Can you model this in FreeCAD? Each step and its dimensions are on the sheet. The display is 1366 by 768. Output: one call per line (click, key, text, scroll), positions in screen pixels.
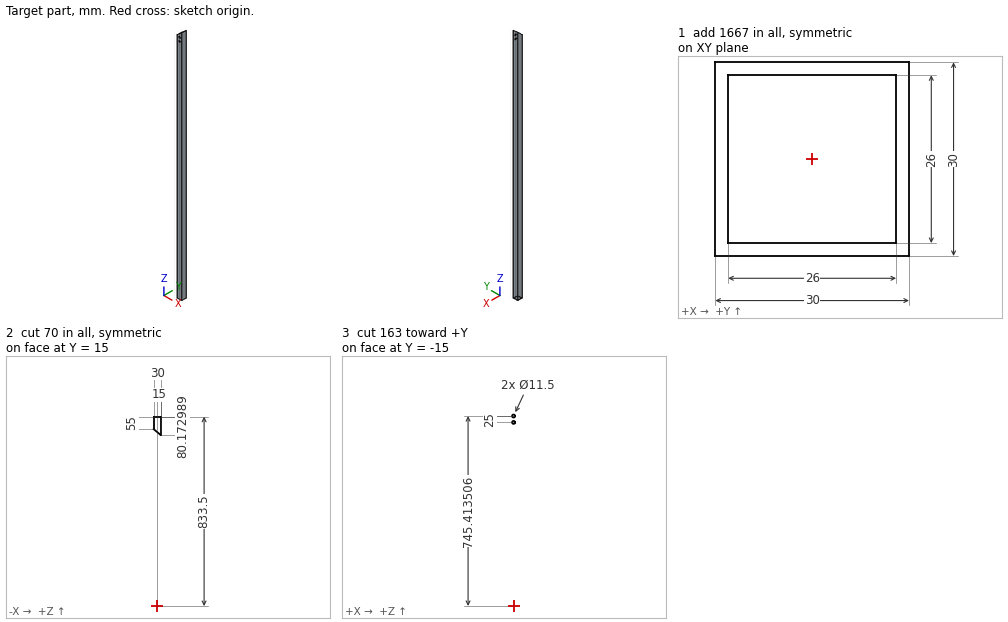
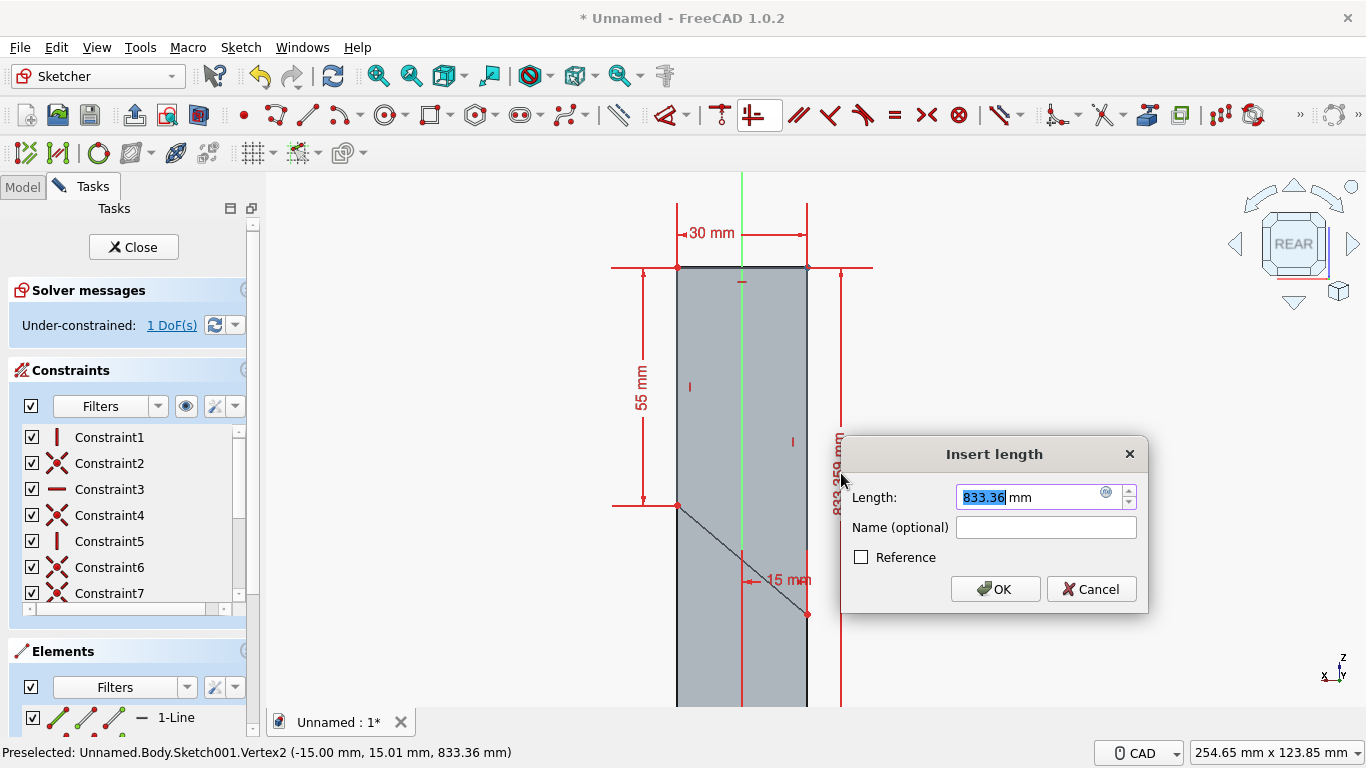
text(833.5)
key(Return)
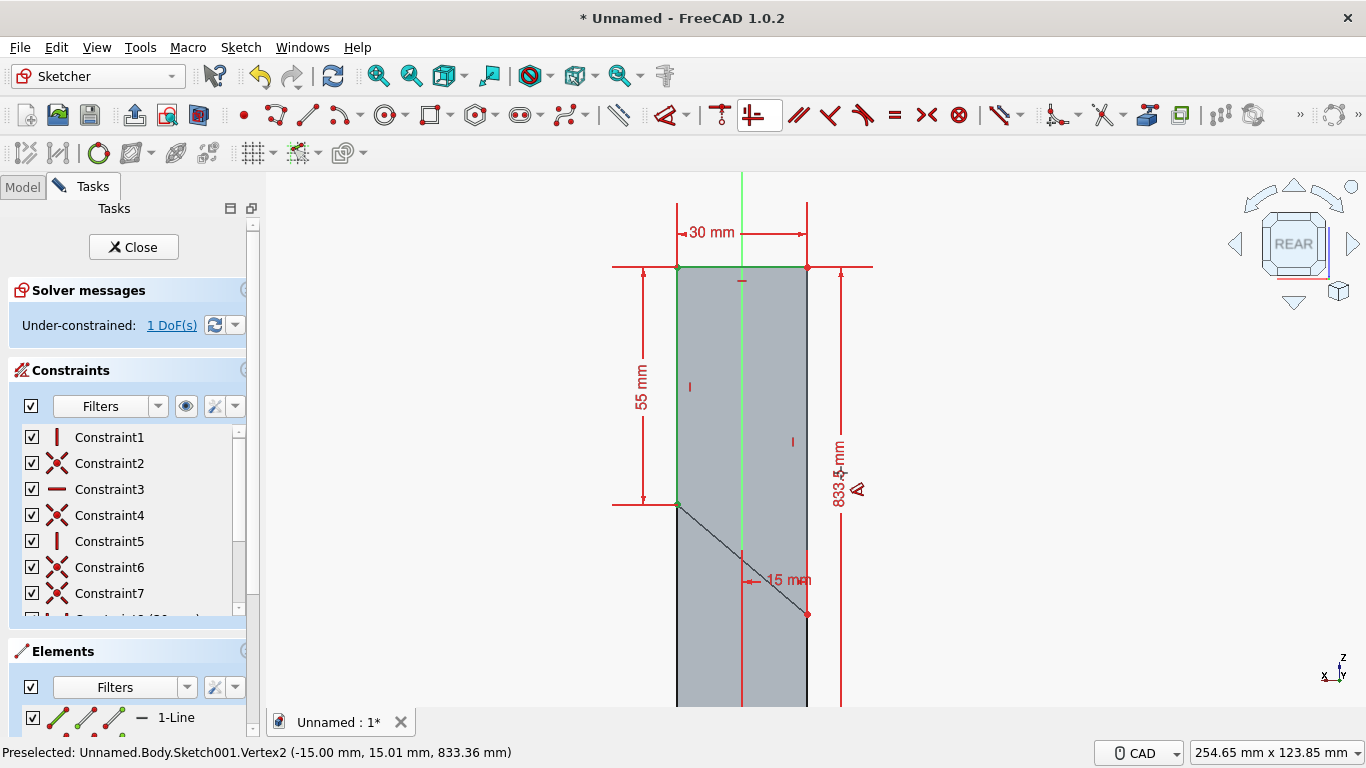
click(807, 511)
click(841, 441)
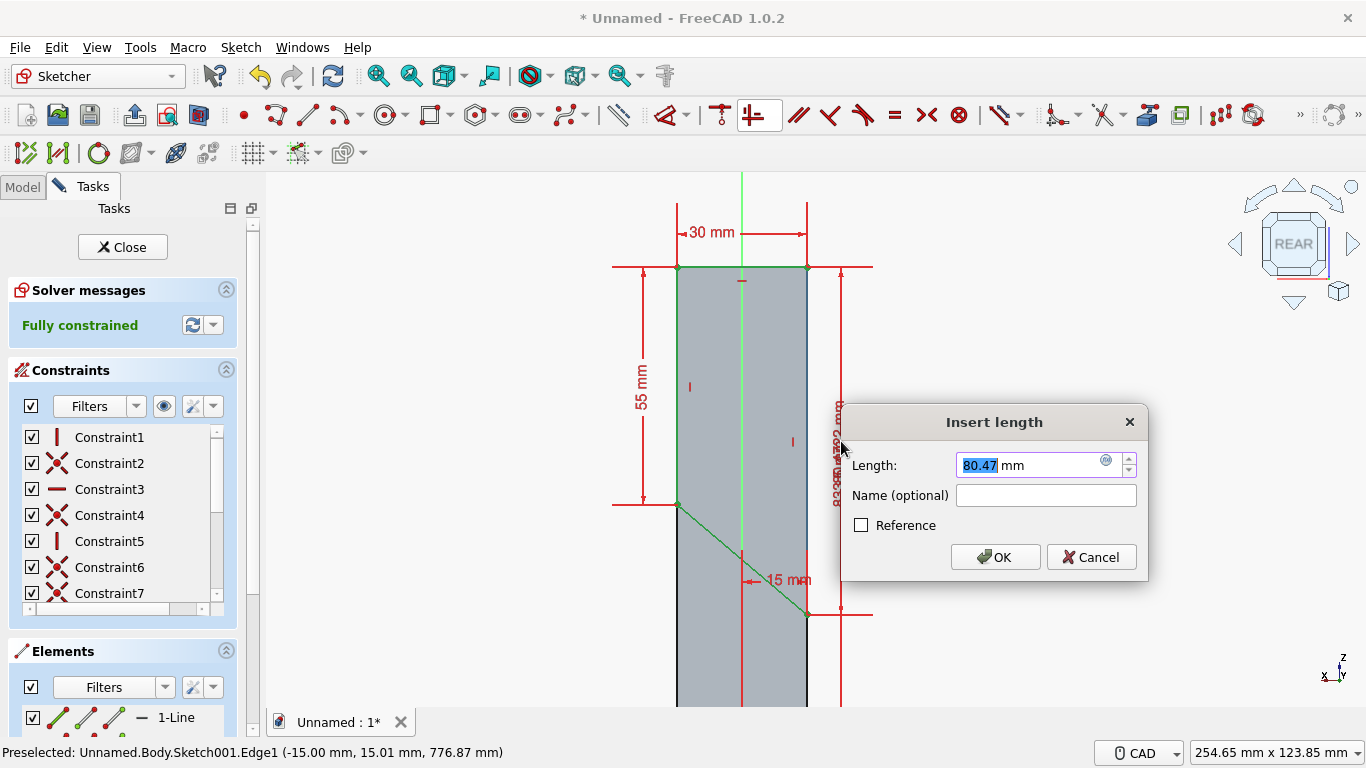
text(80.172989)
key(Return)
key(Escape)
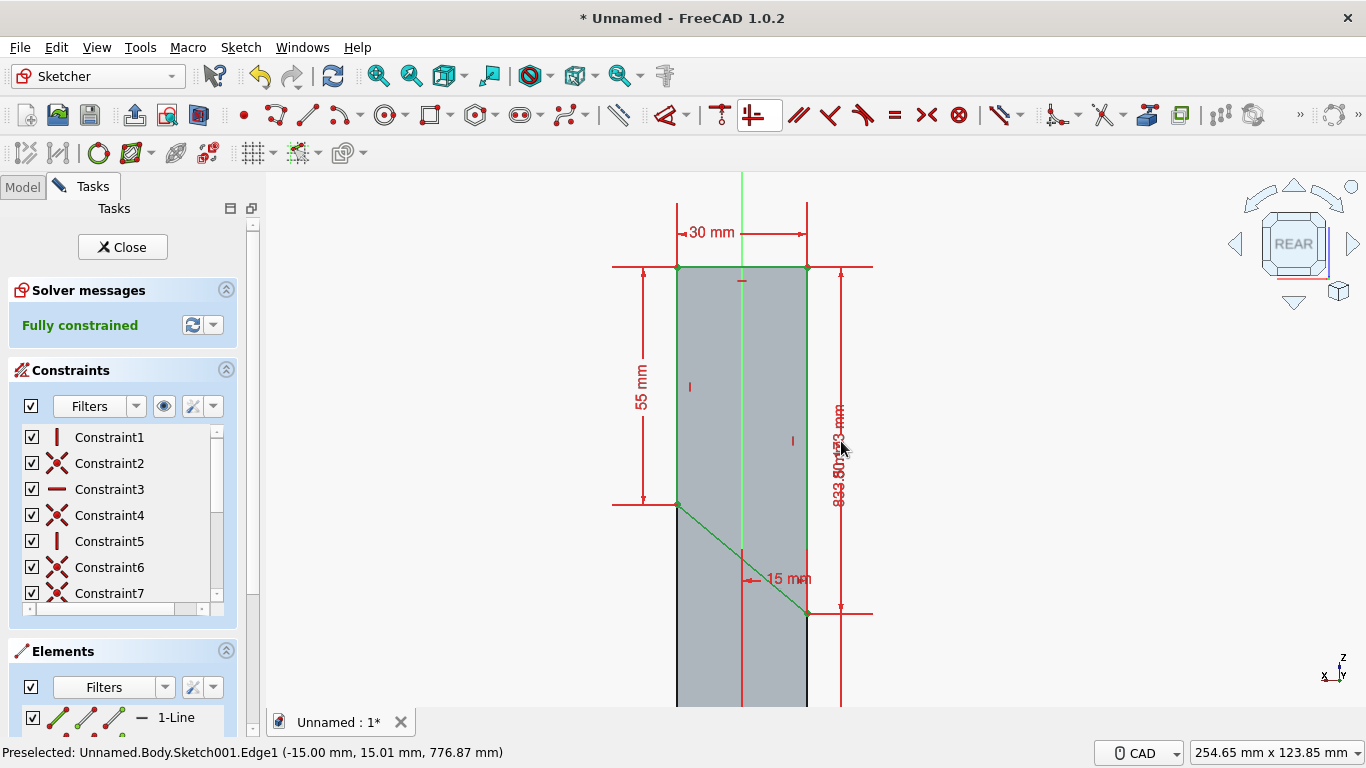
click(123, 247)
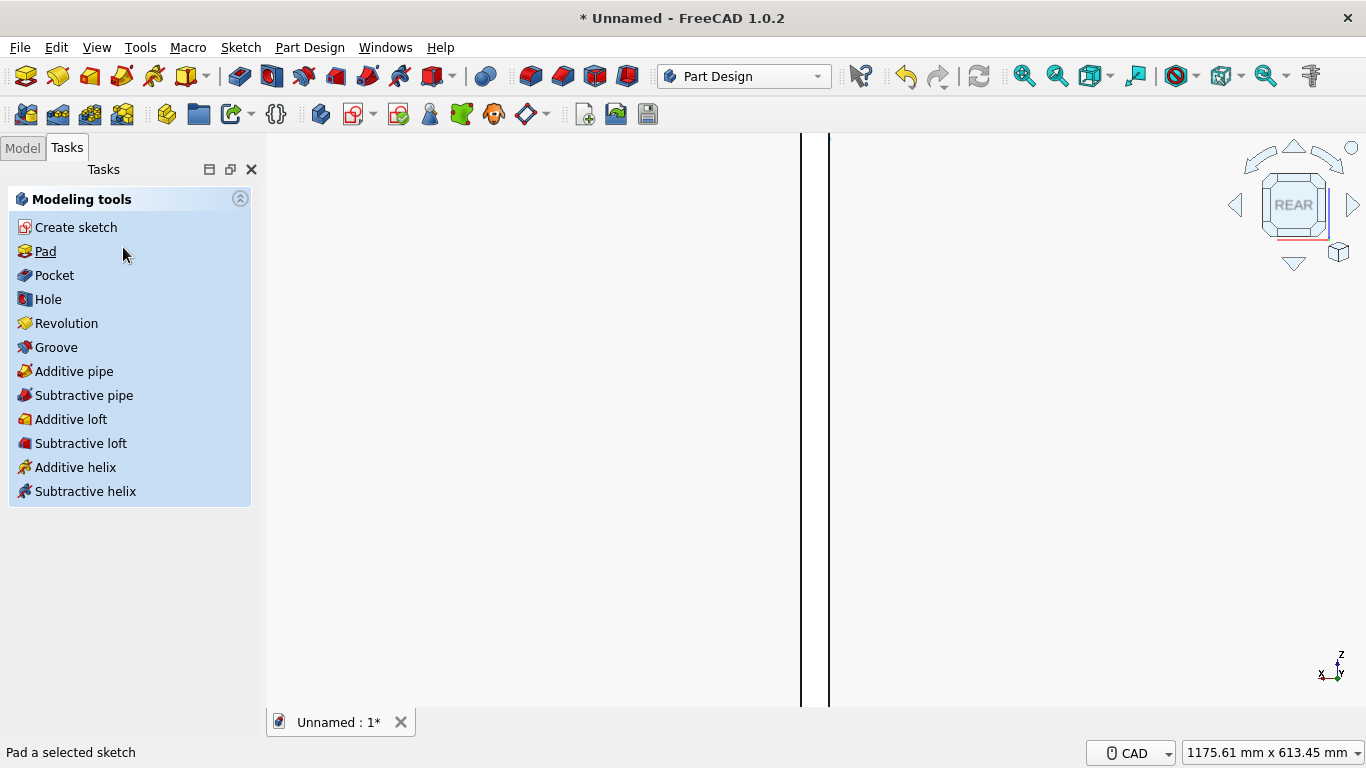
click(240, 76)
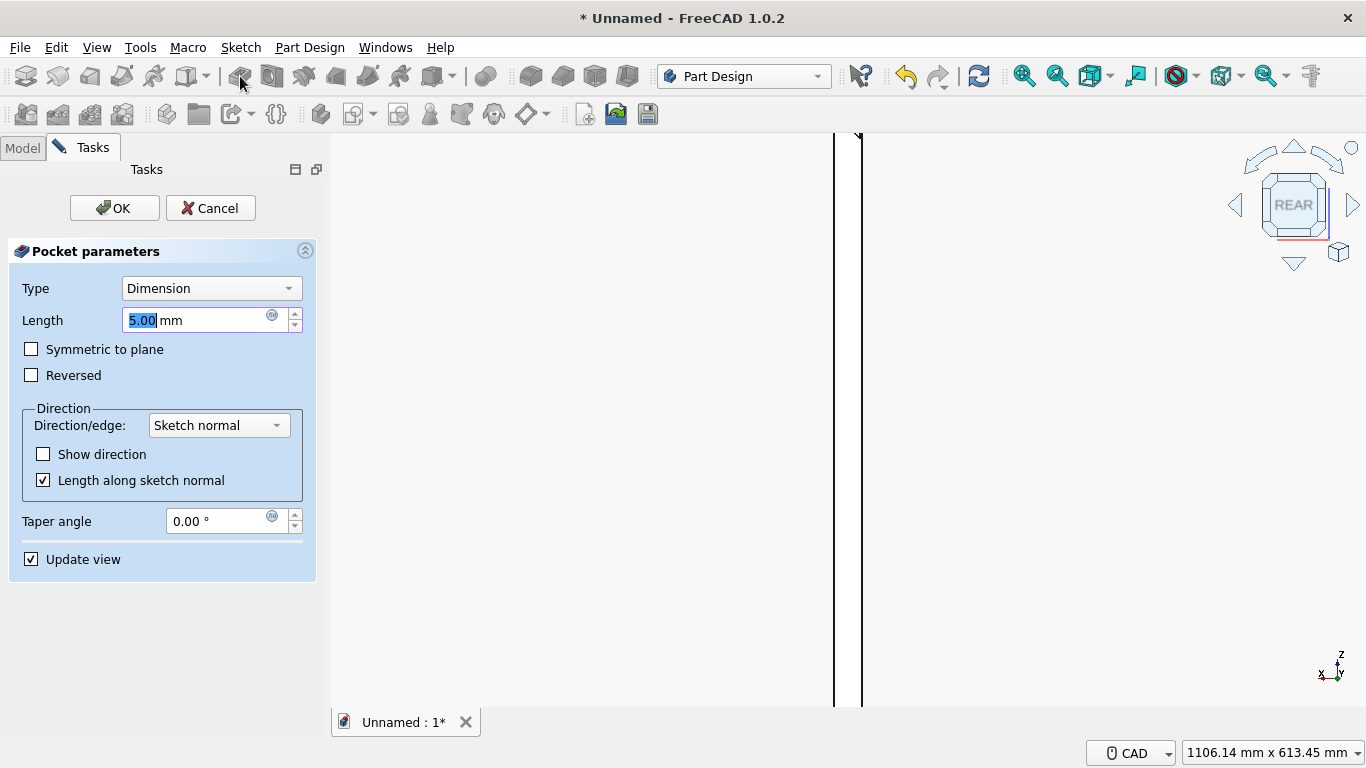
text(70)
key(Tab)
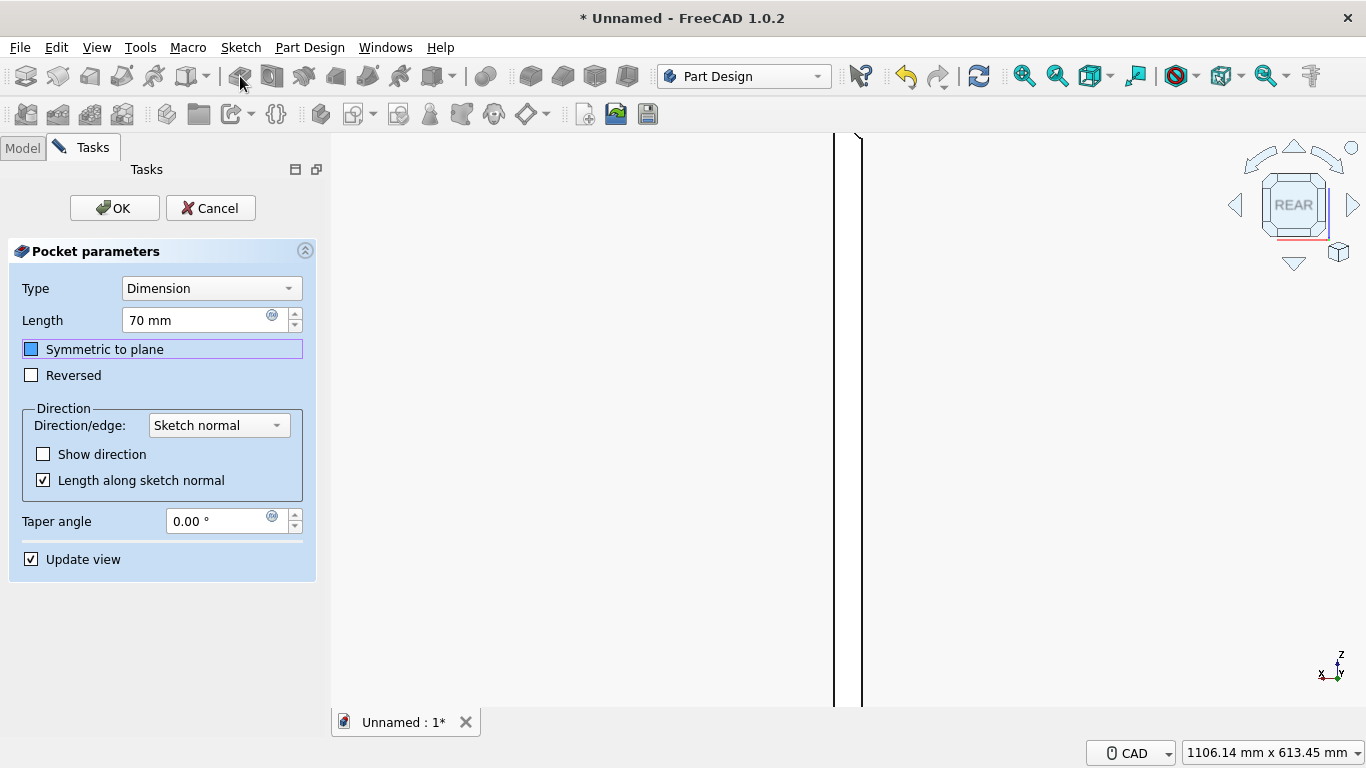
click(30, 349)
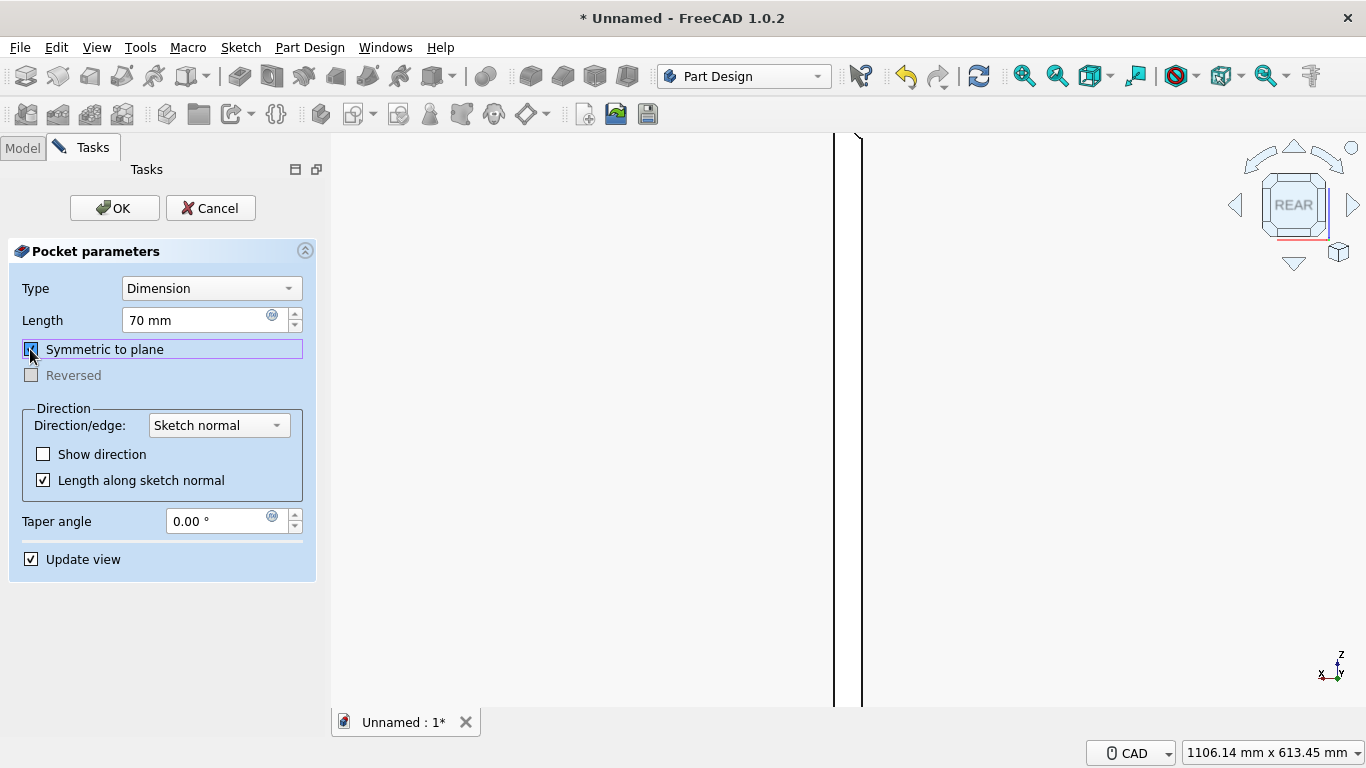
click(115, 208)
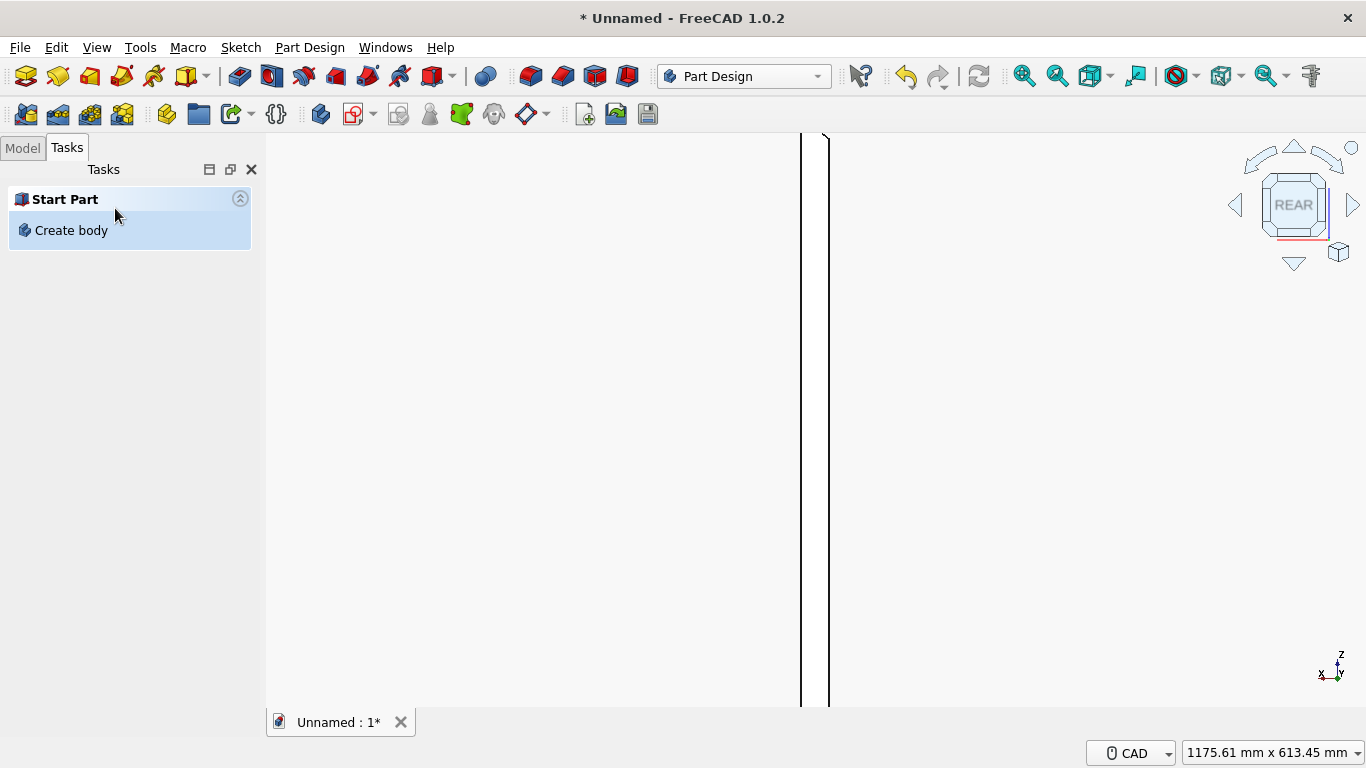
key(v)
key(f)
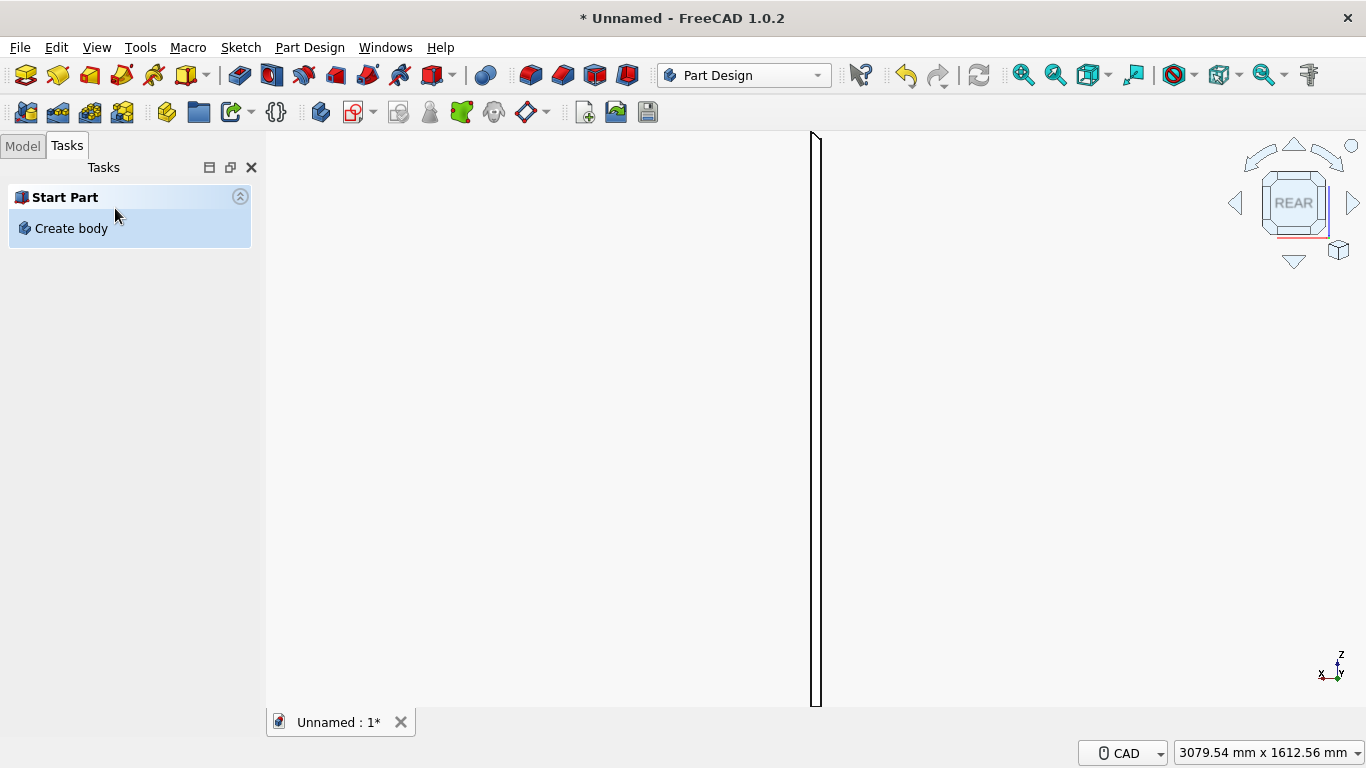
key(0)